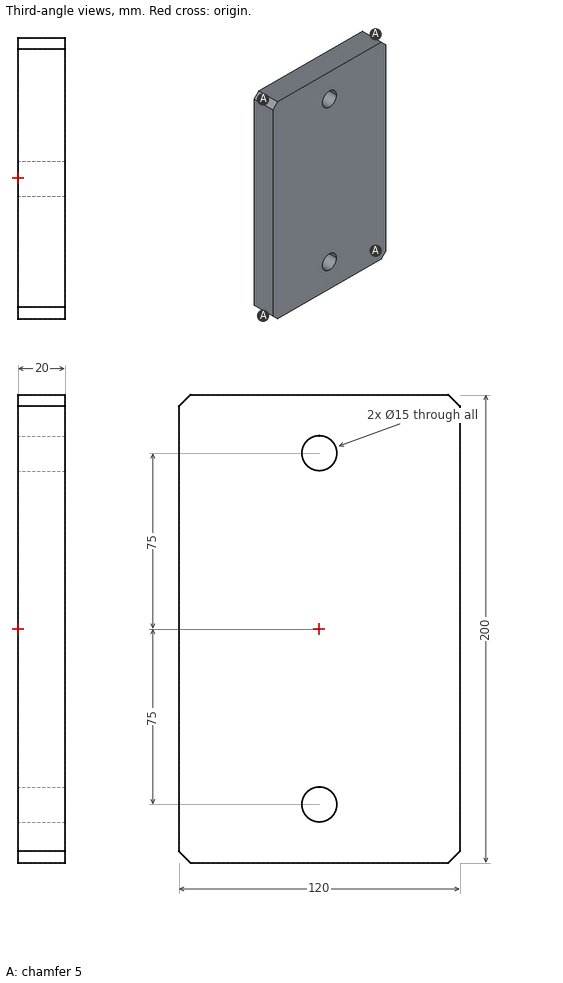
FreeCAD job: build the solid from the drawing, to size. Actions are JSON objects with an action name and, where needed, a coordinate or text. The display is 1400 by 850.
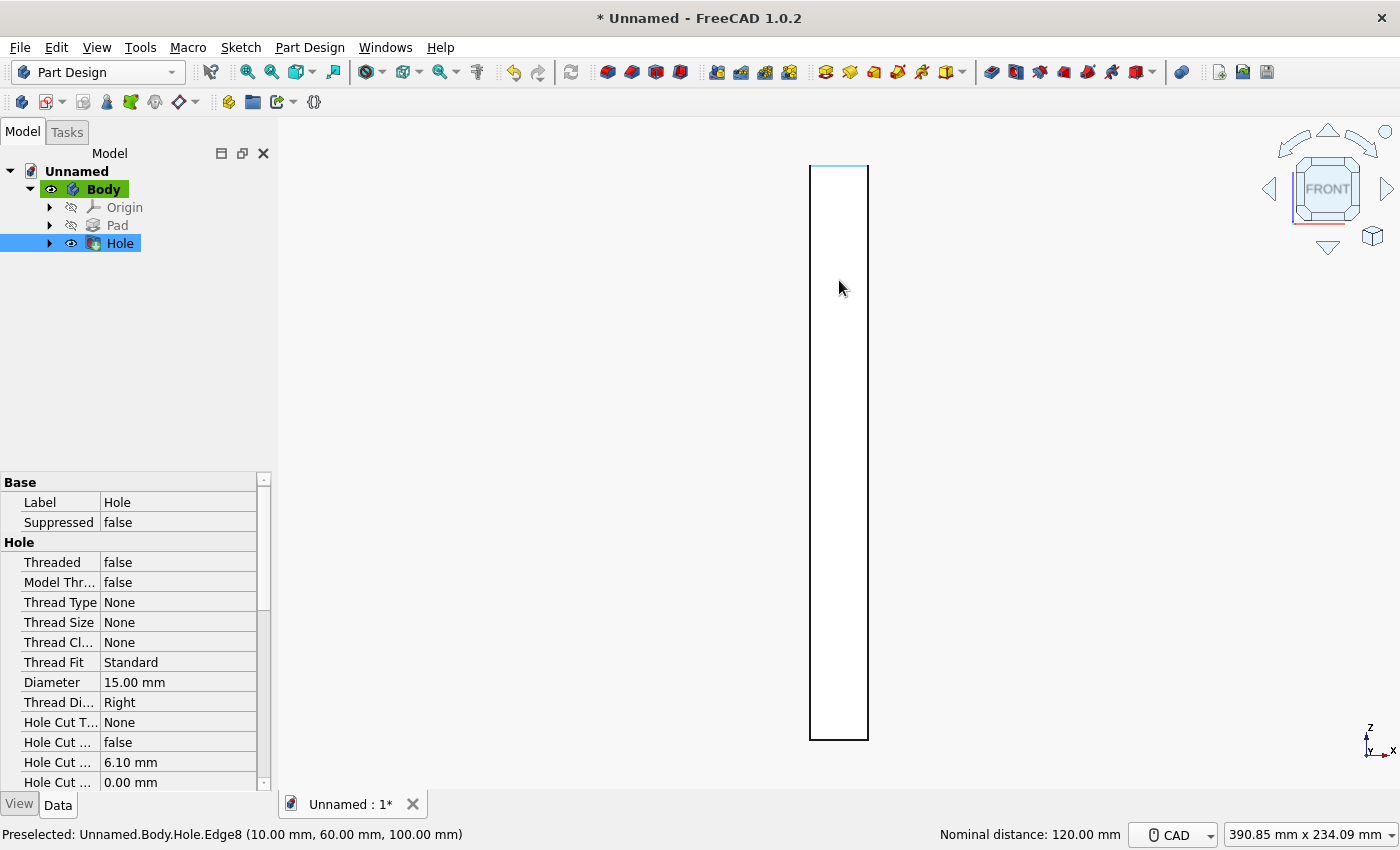
{"action": "left_click", "coordinate": [839, 739], "text": "ctrl"}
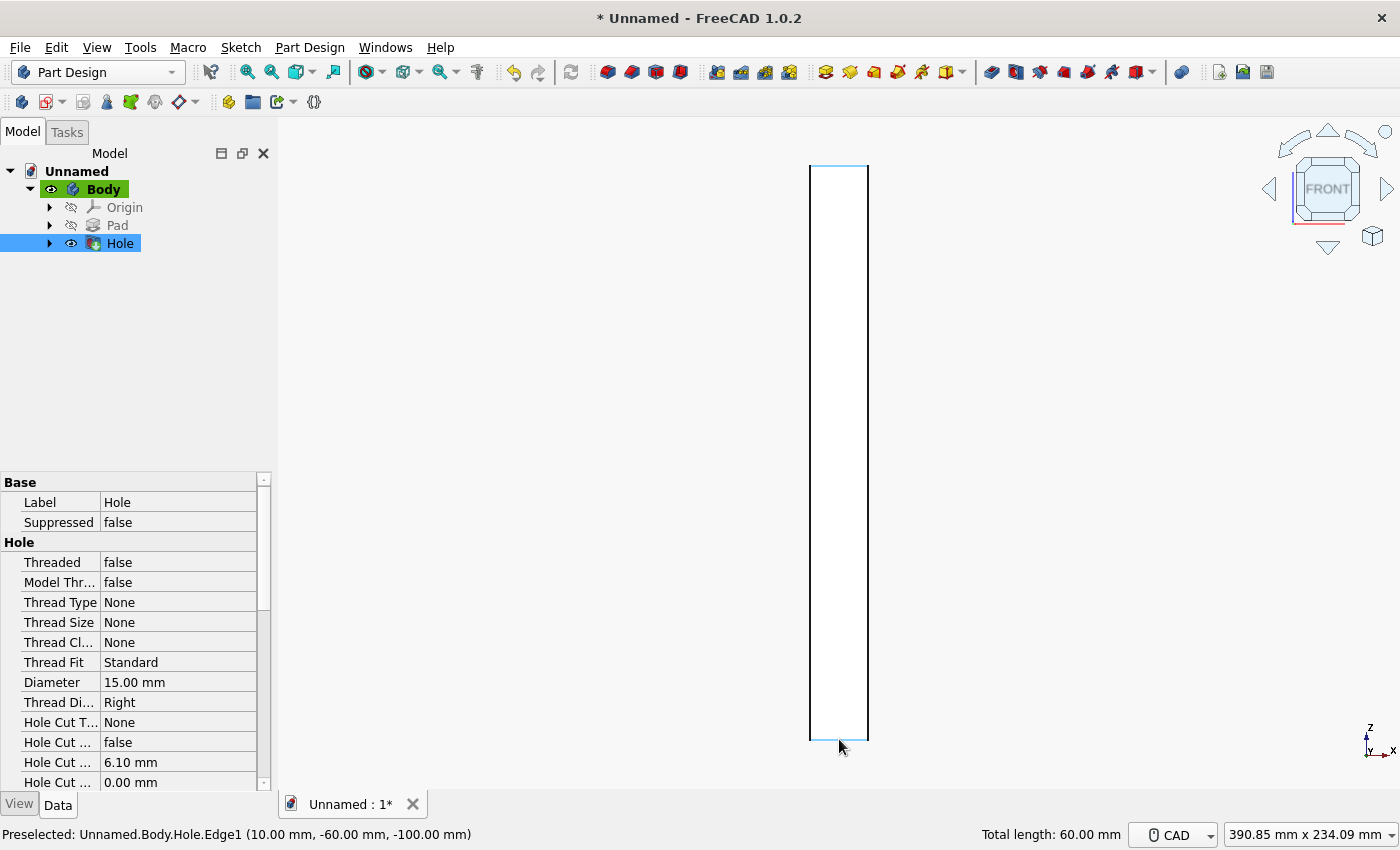
{"action": "key", "text": "3"}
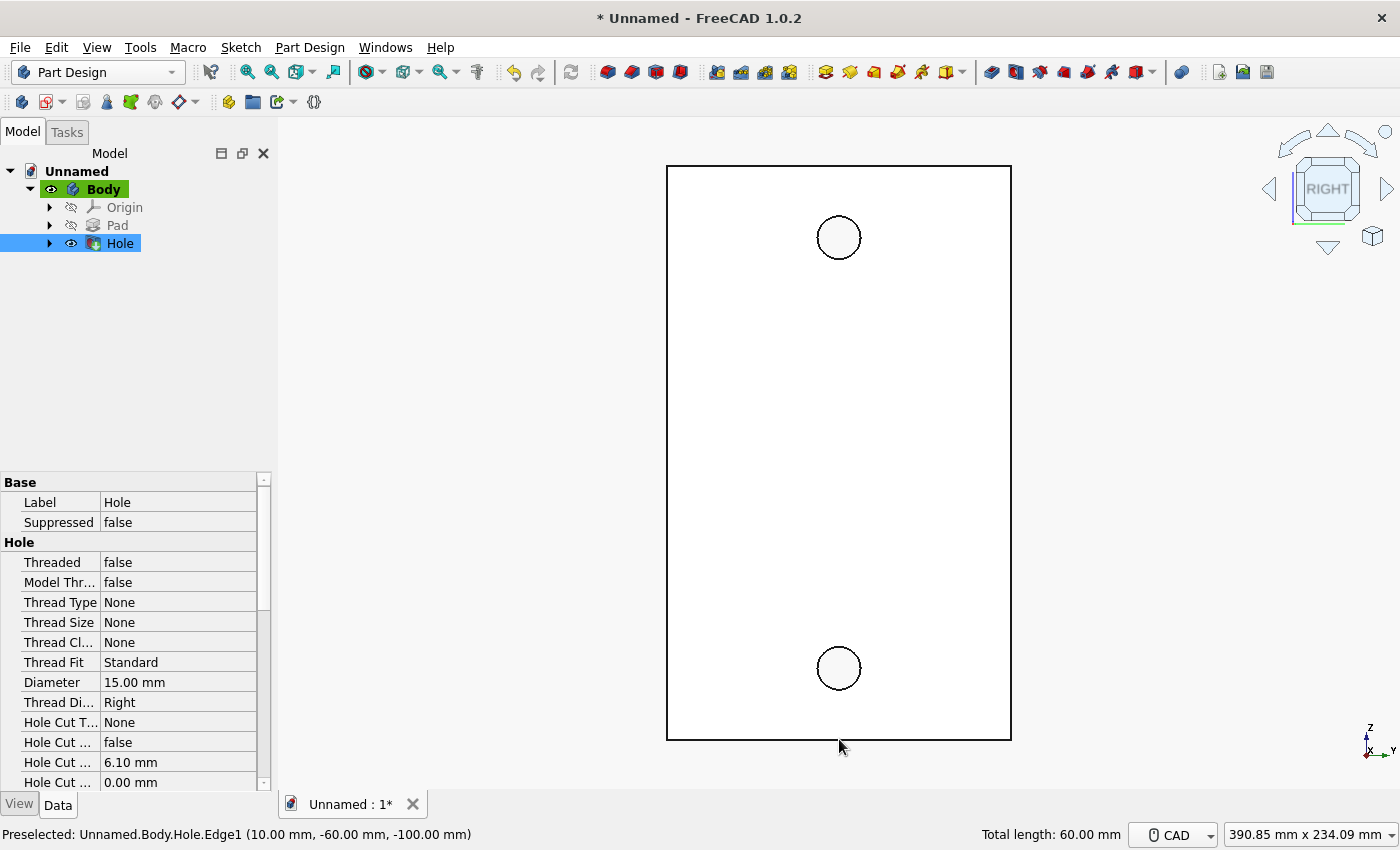
{"action": "key", "text": "5"}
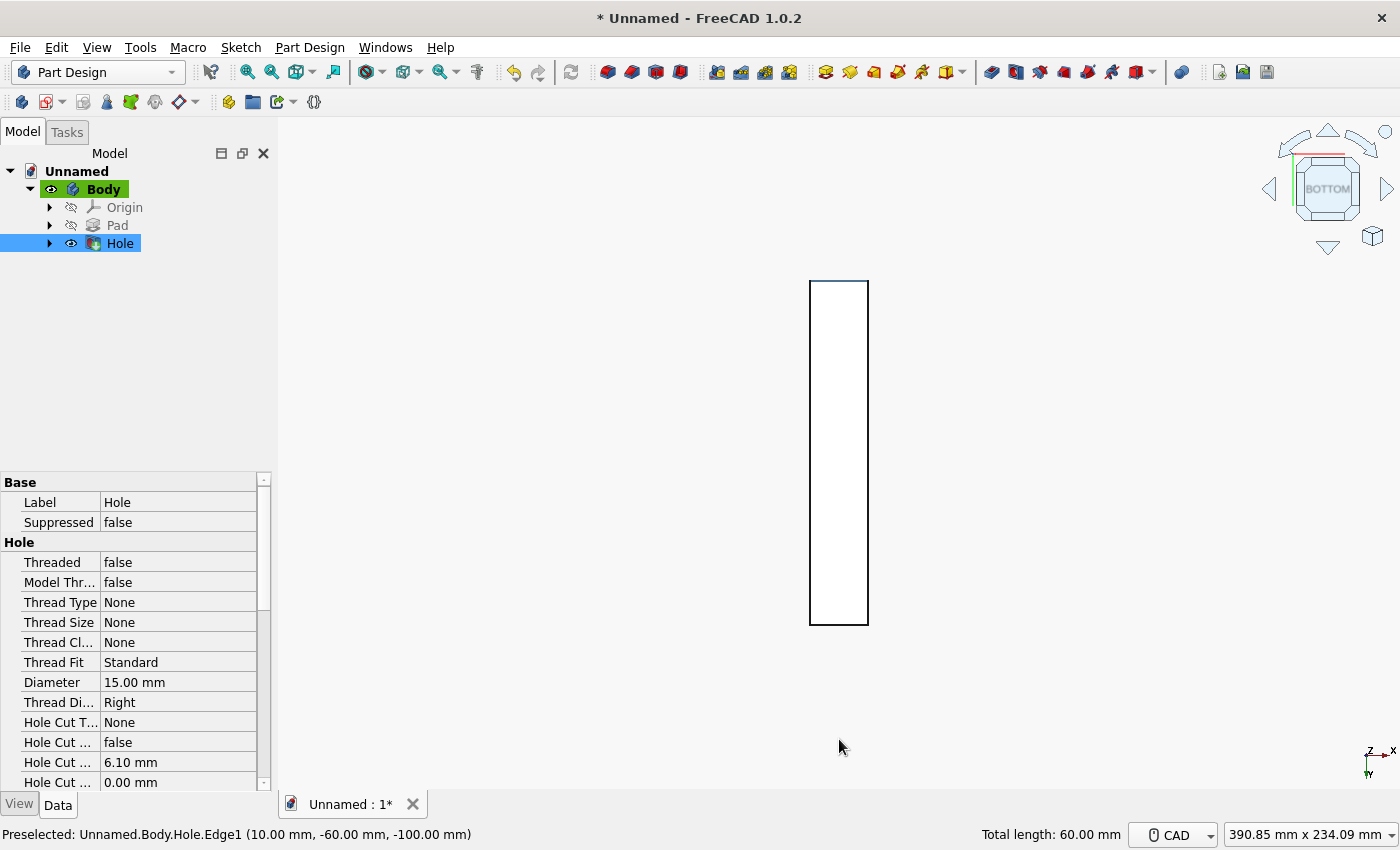
{"action": "left_click", "coordinate": [839, 624], "text": "ctrl"}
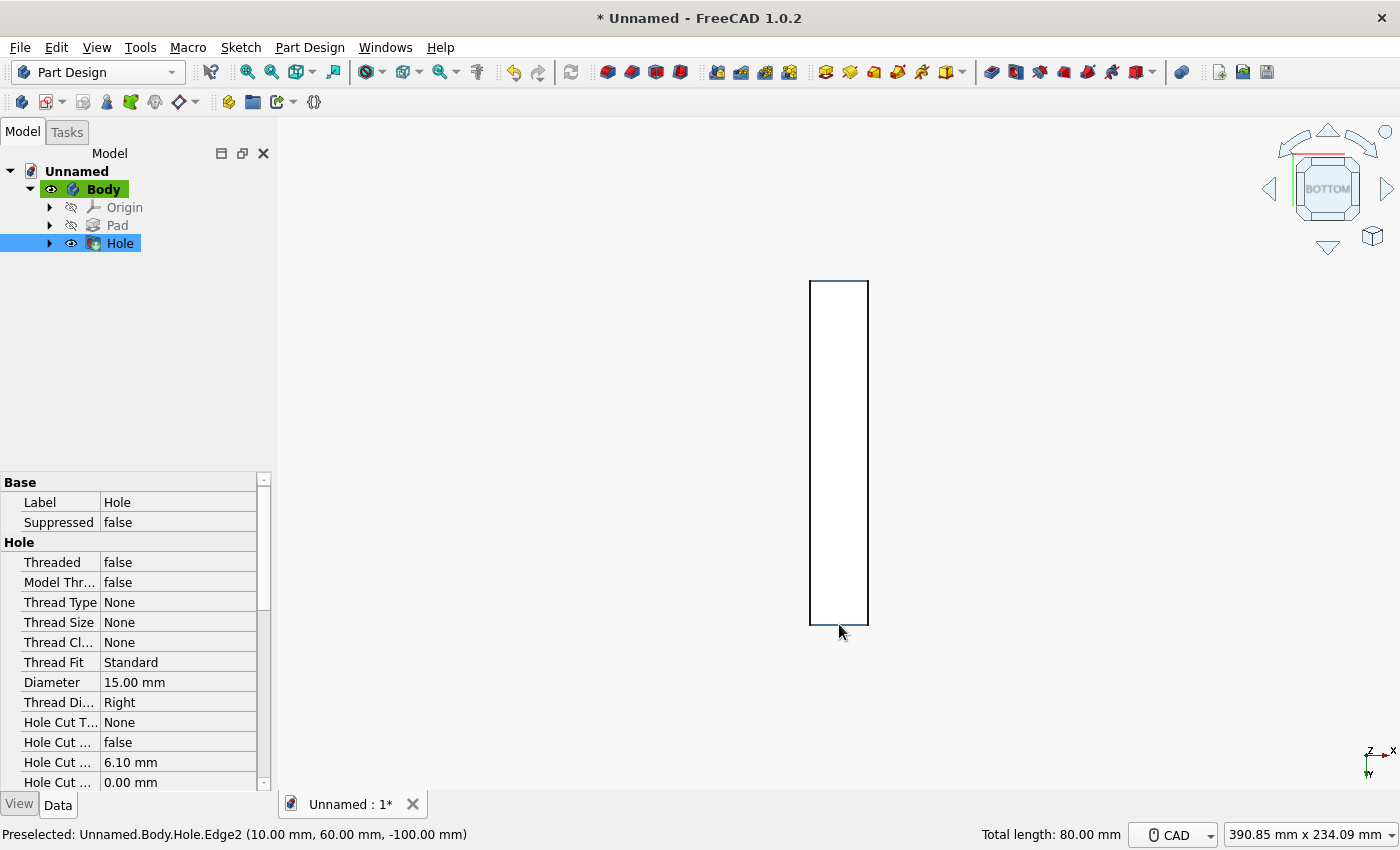
{"action": "left_click", "coordinate": [632, 72]}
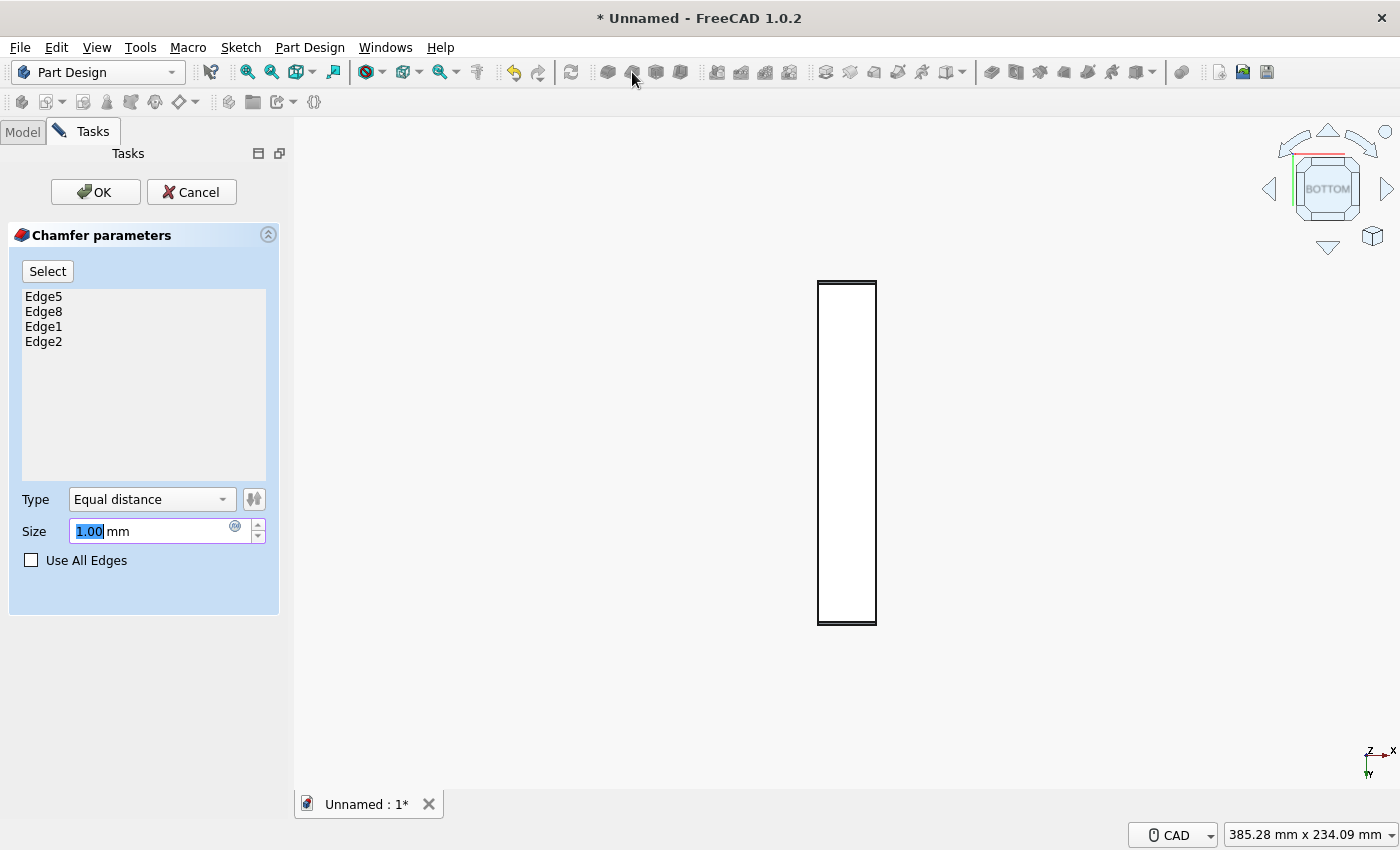
{"action": "type", "text": "5"}
{"action": "key", "text": "Tab"}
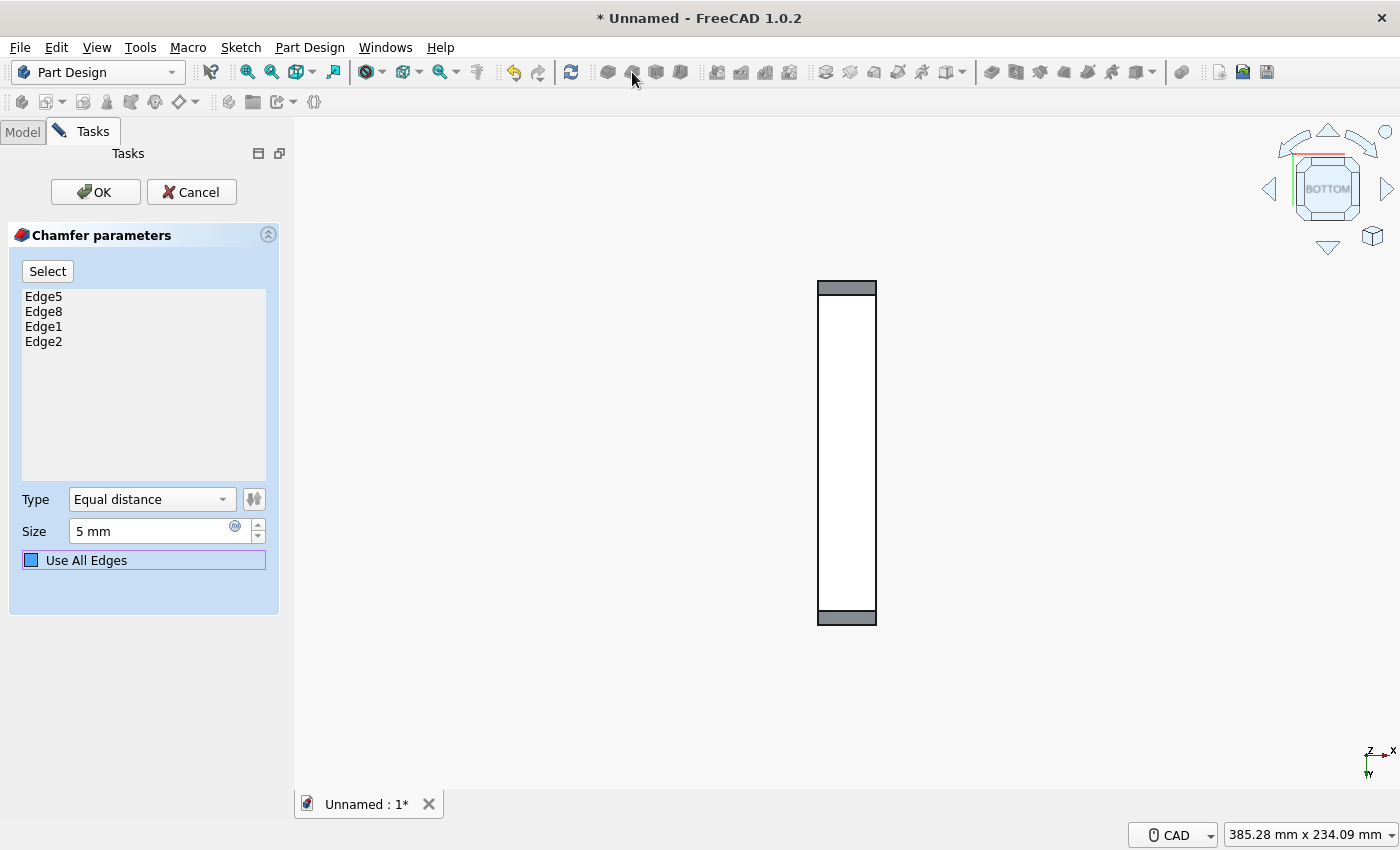
{"action": "left_click", "coordinate": [96, 192]}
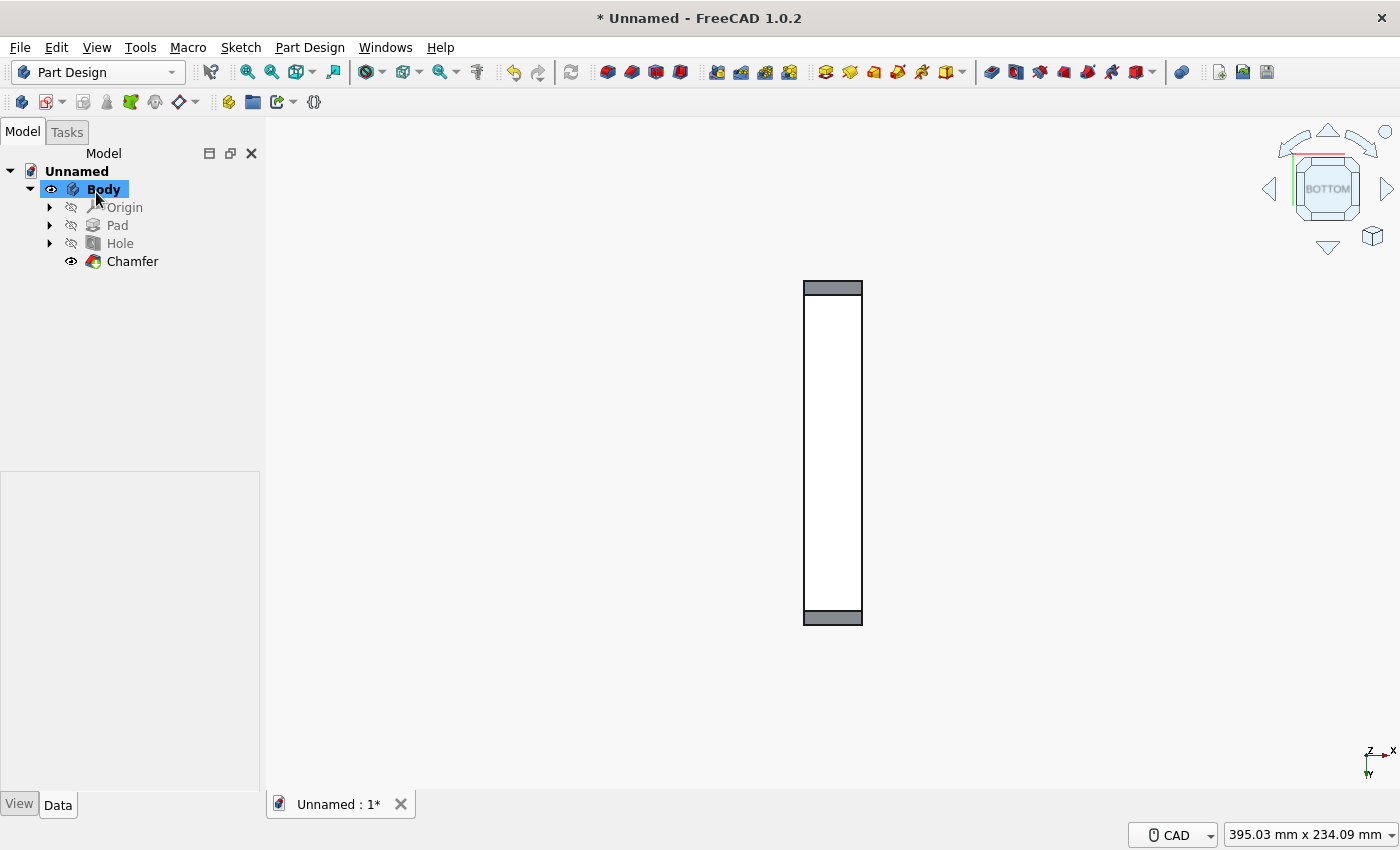
{"action": "key", "text": "0"}